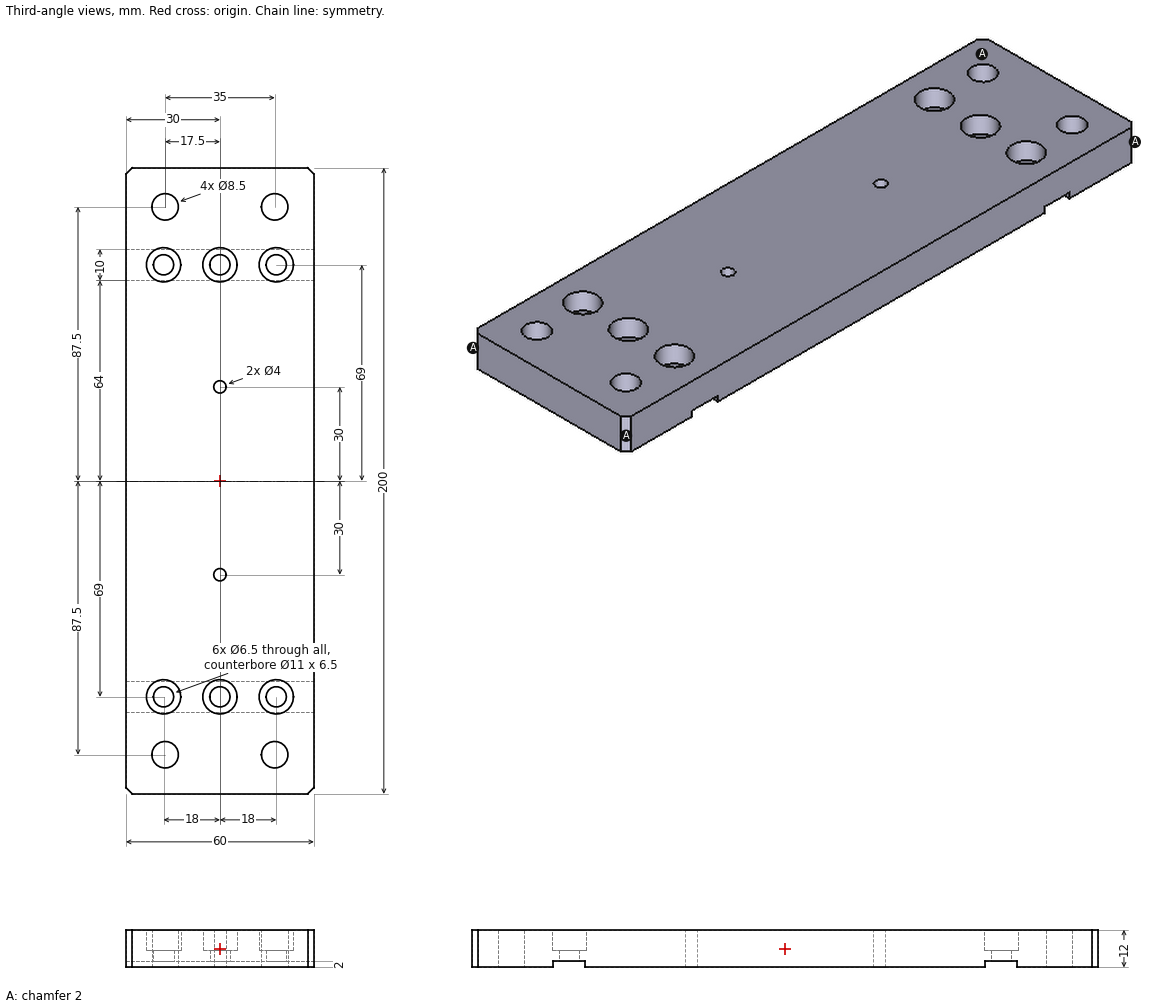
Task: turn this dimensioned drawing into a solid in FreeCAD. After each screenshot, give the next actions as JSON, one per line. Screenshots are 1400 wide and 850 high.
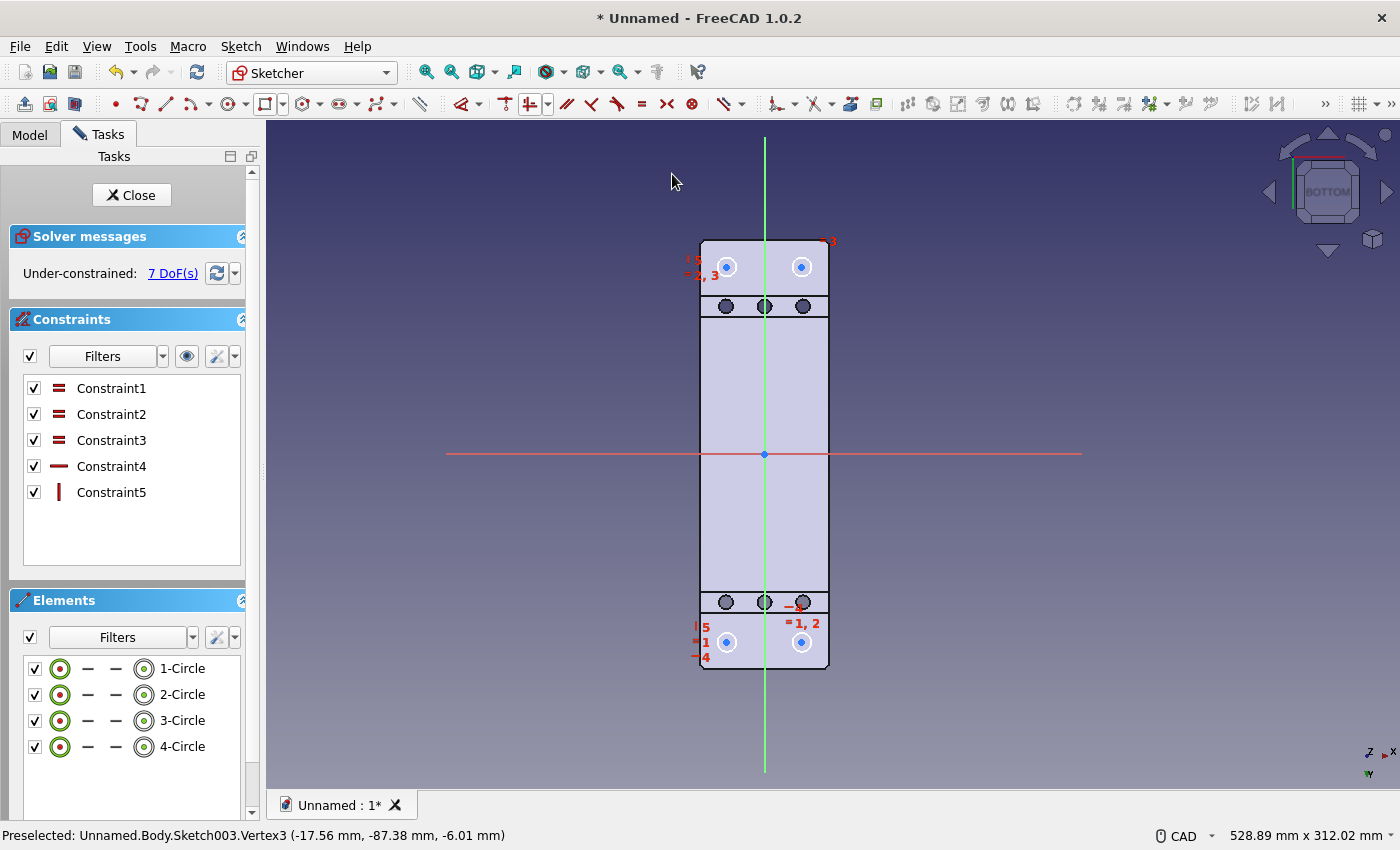
{"action": "left_click", "coordinate": [802, 642]}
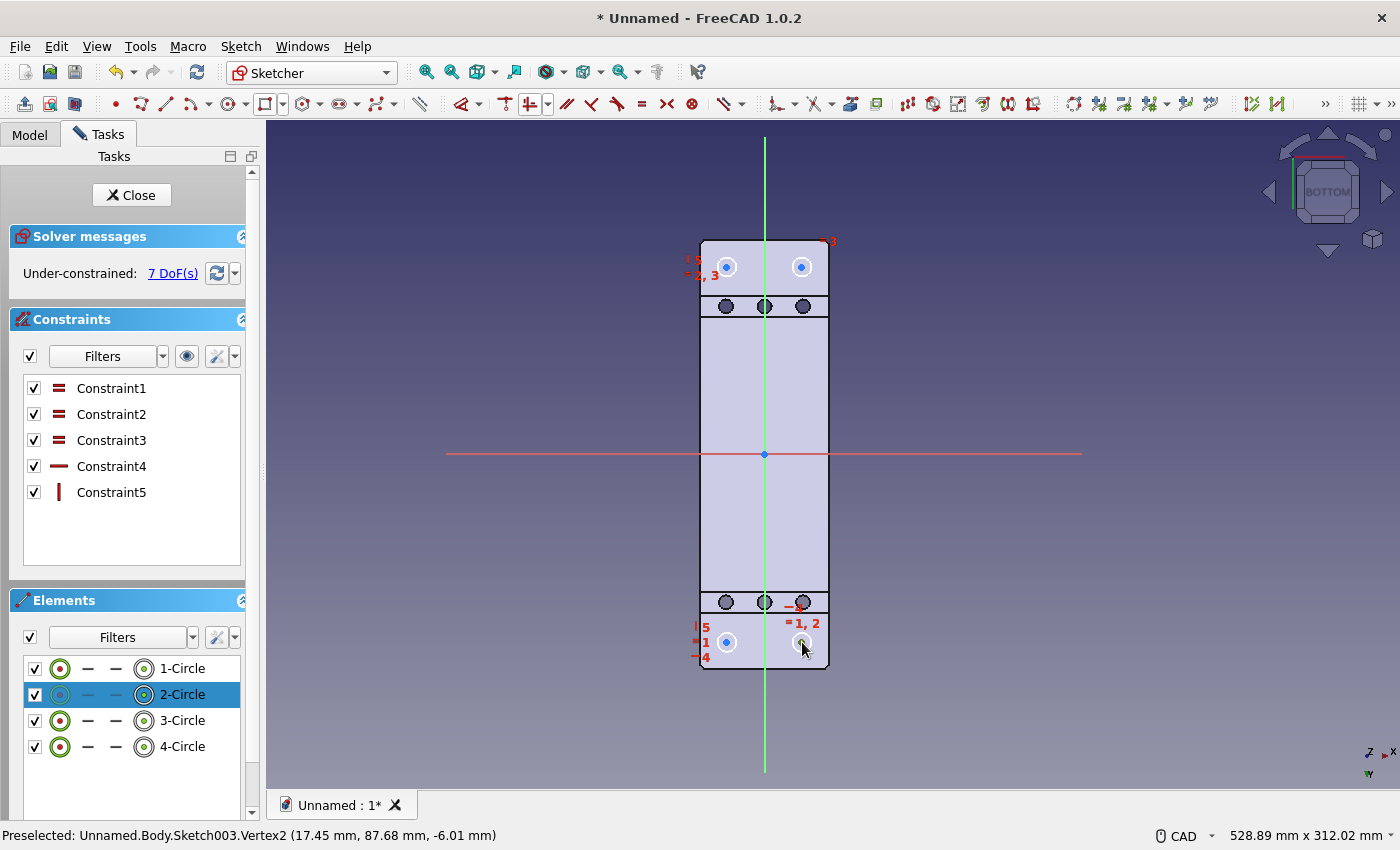
{"action": "left_click", "coordinate": [802, 267]}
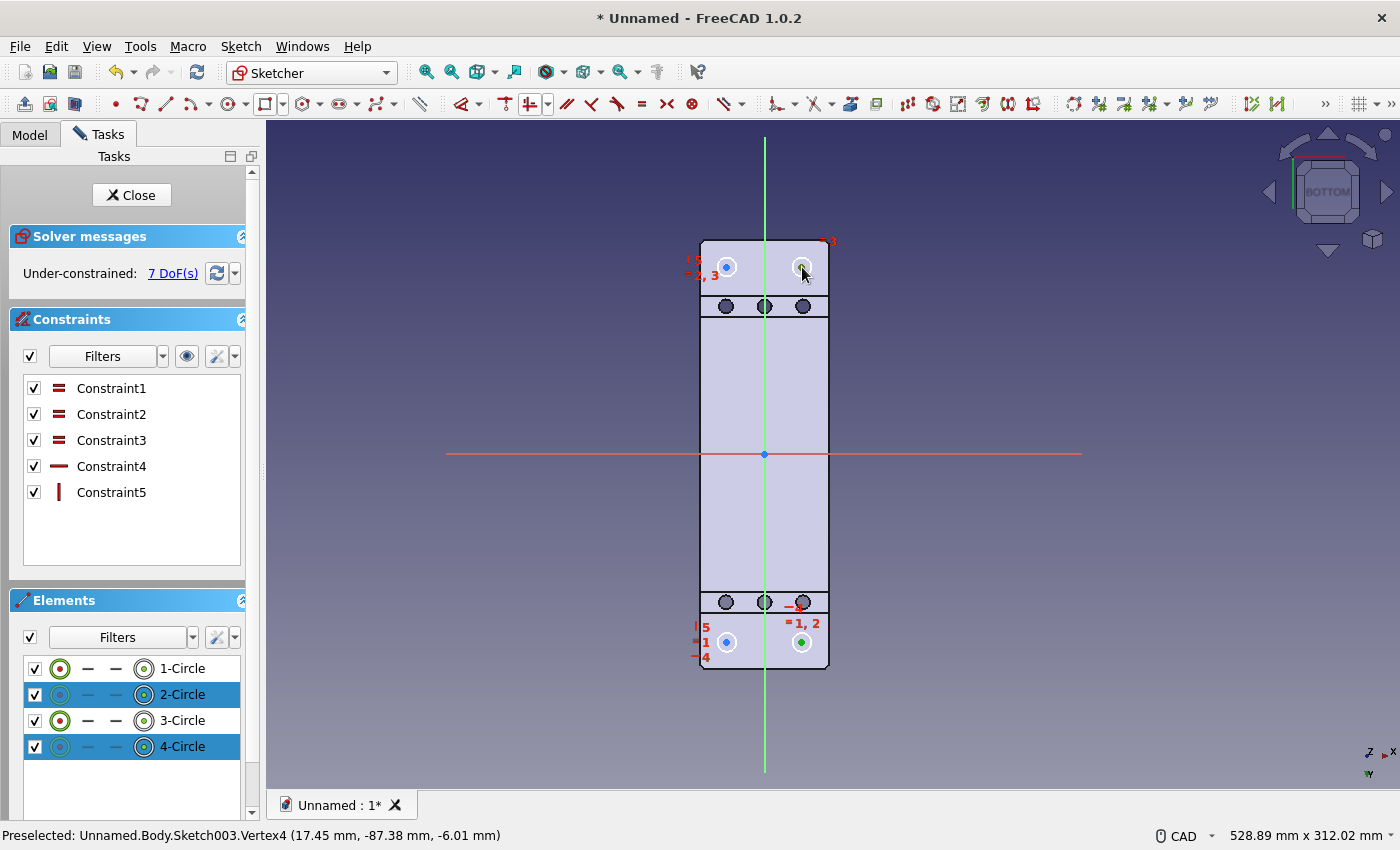
{"action": "key", "text": "v"}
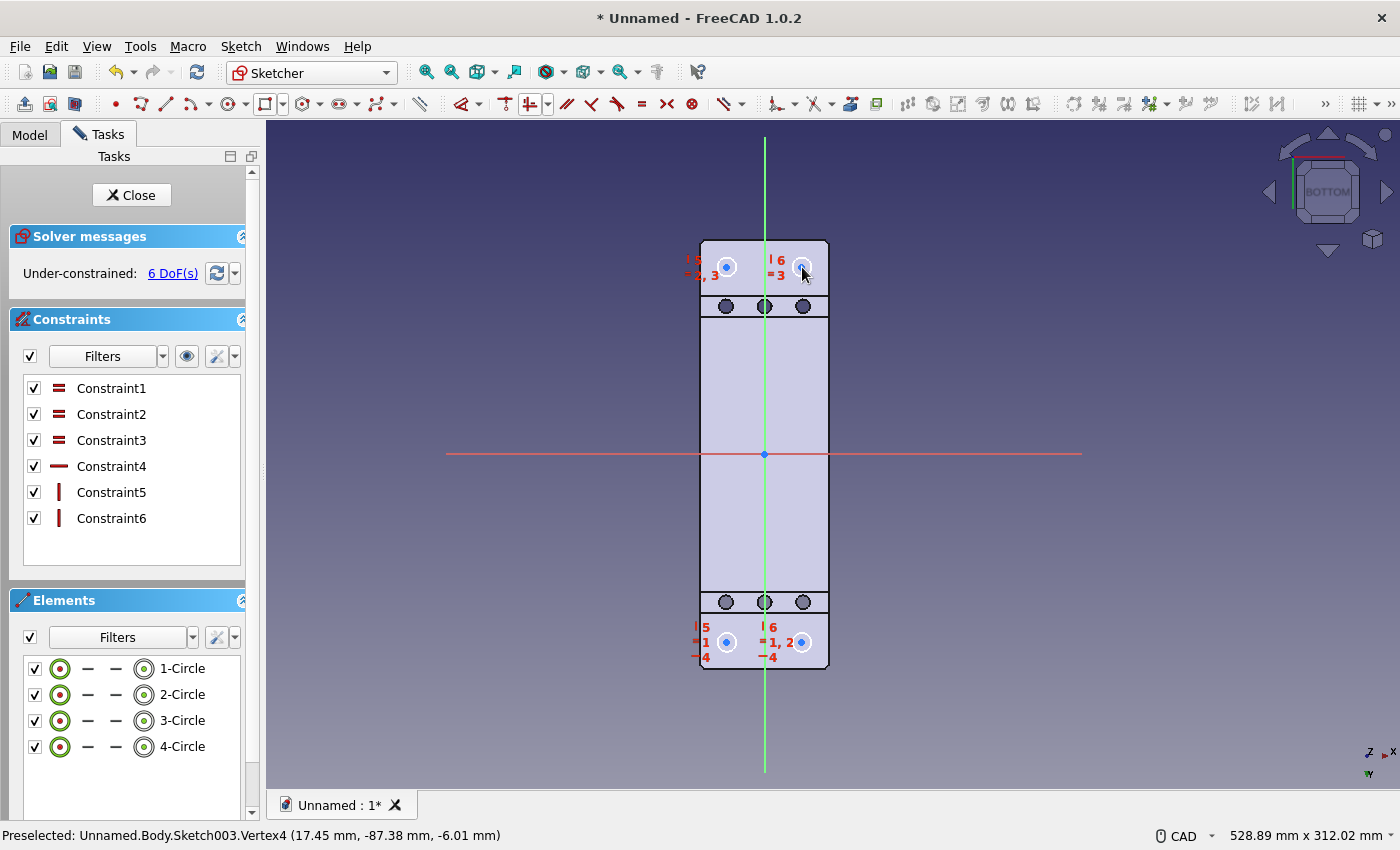
{"action": "left_click", "coordinate": [727, 267]}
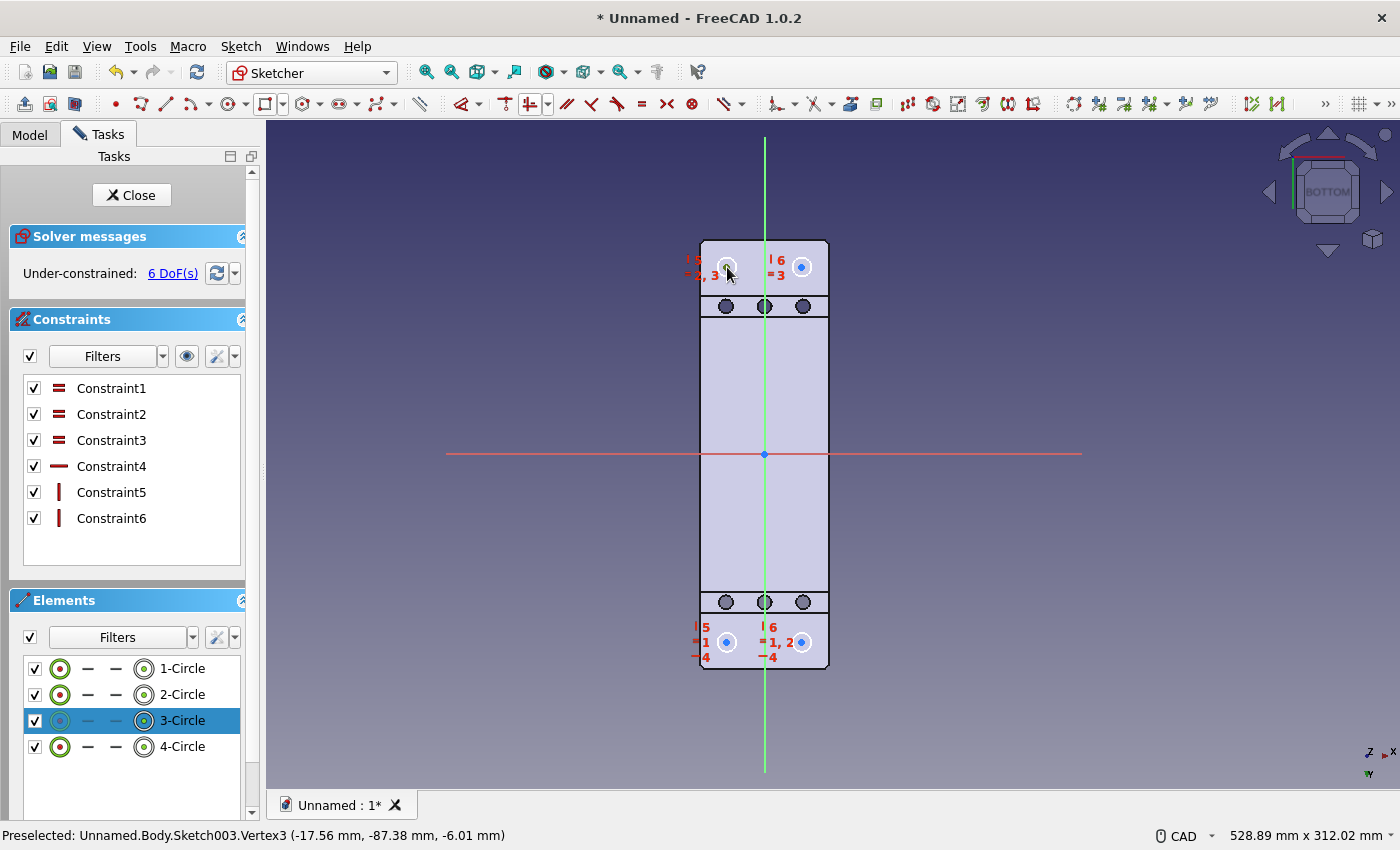
{"action": "left_click", "coordinate": [802, 267]}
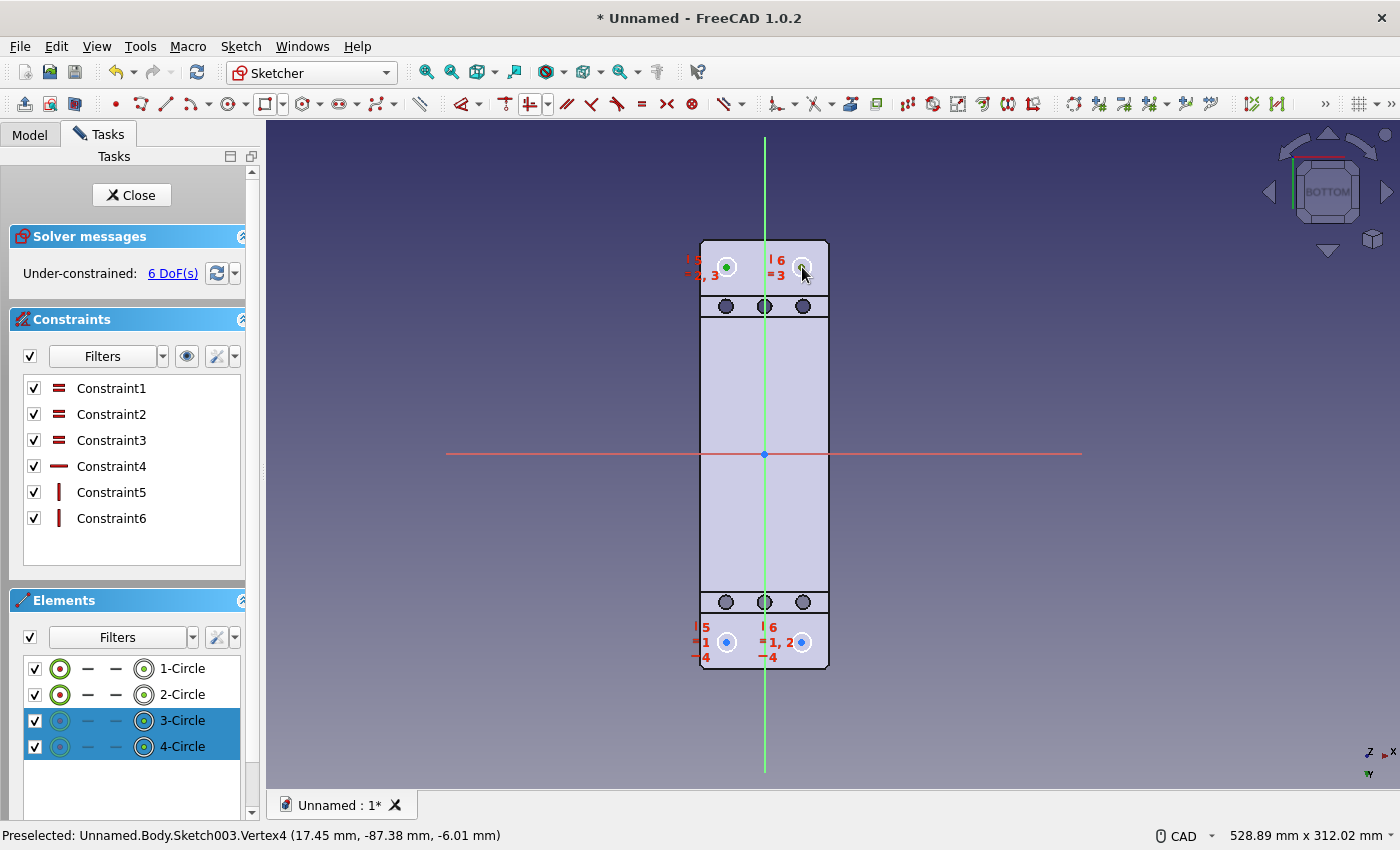
{"action": "left_click", "coordinate": [548, 104]}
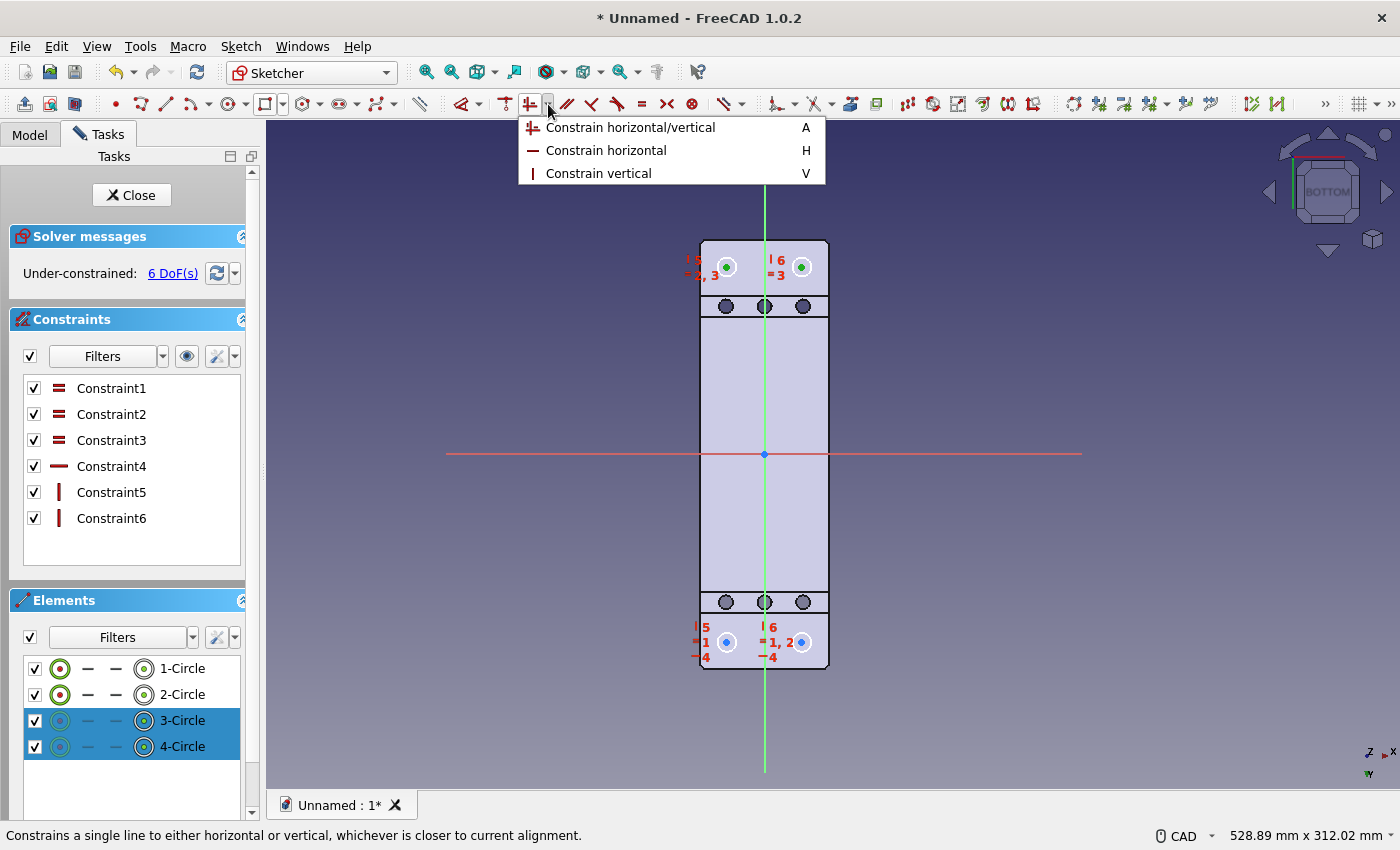
{"action": "left_click", "coordinate": [672, 150]}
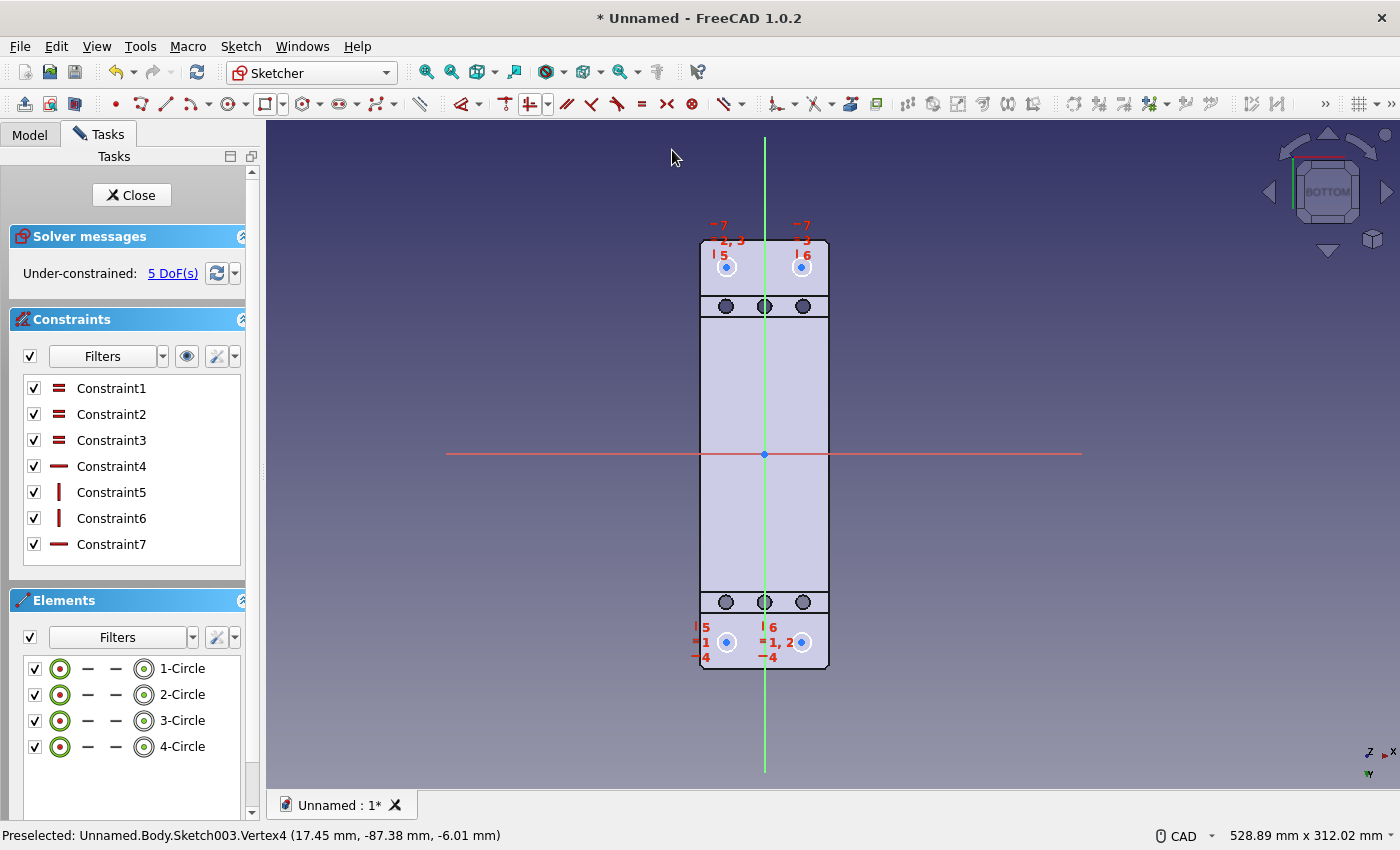
{"action": "left_click", "coordinate": [460, 104]}